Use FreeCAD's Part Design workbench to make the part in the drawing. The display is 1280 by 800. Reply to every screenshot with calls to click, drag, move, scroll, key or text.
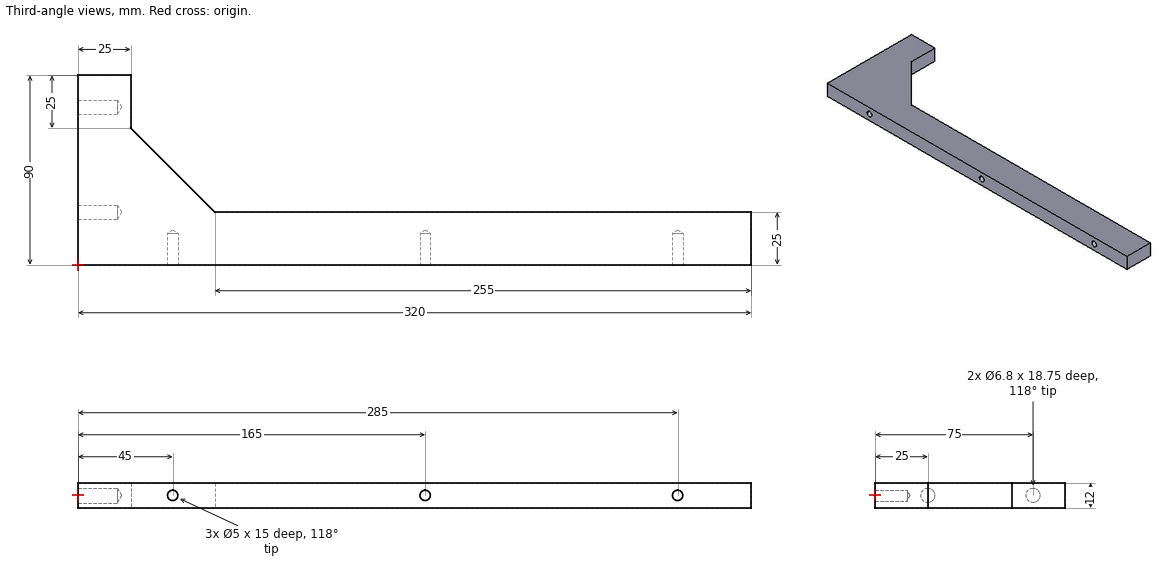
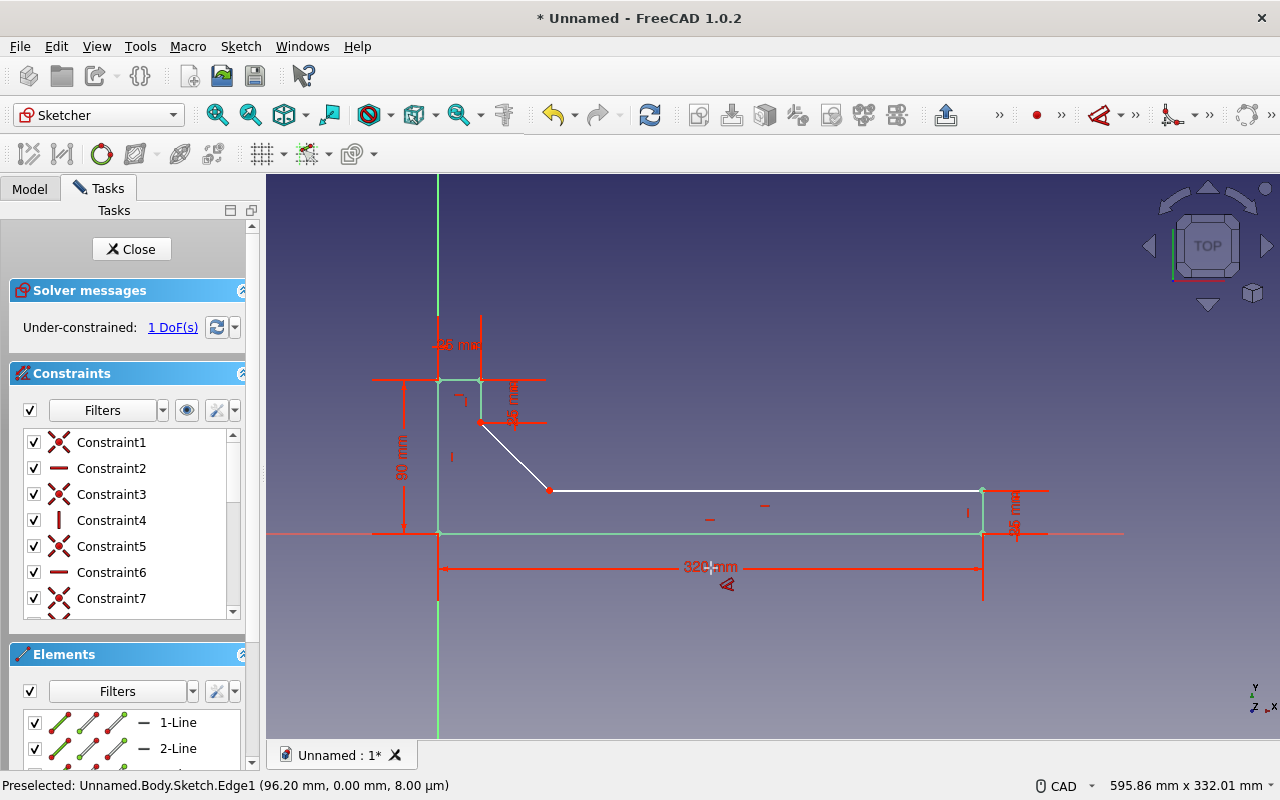
click(853, 491)
click(766, 457)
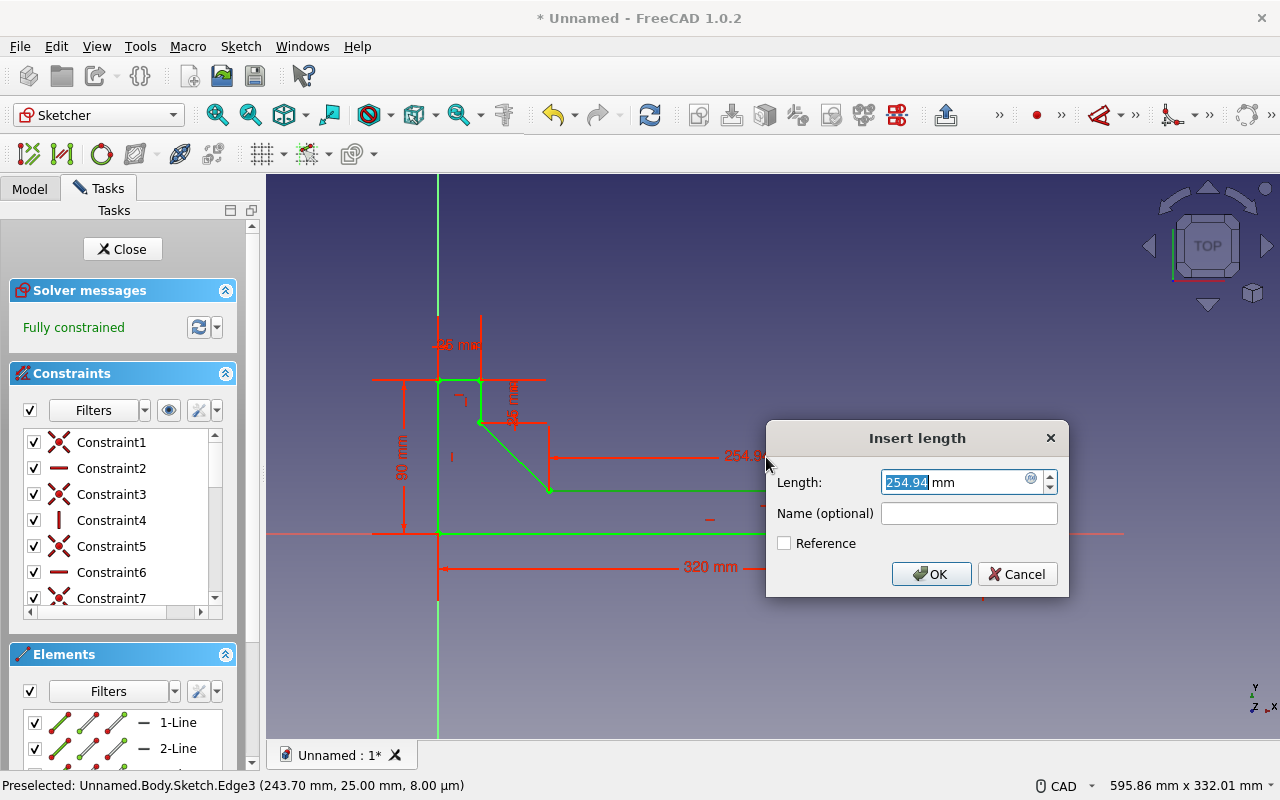
text(255)
key(Return)
key(Escape)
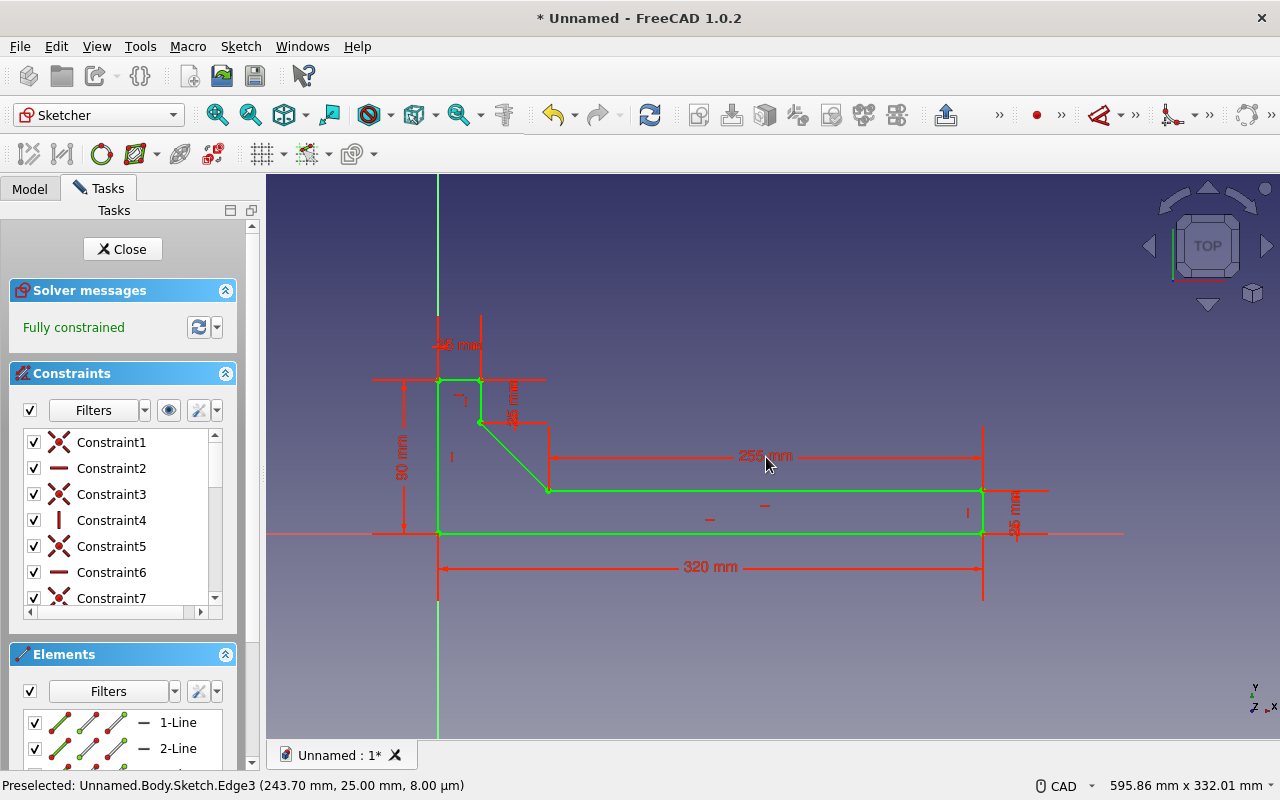
click(123, 249)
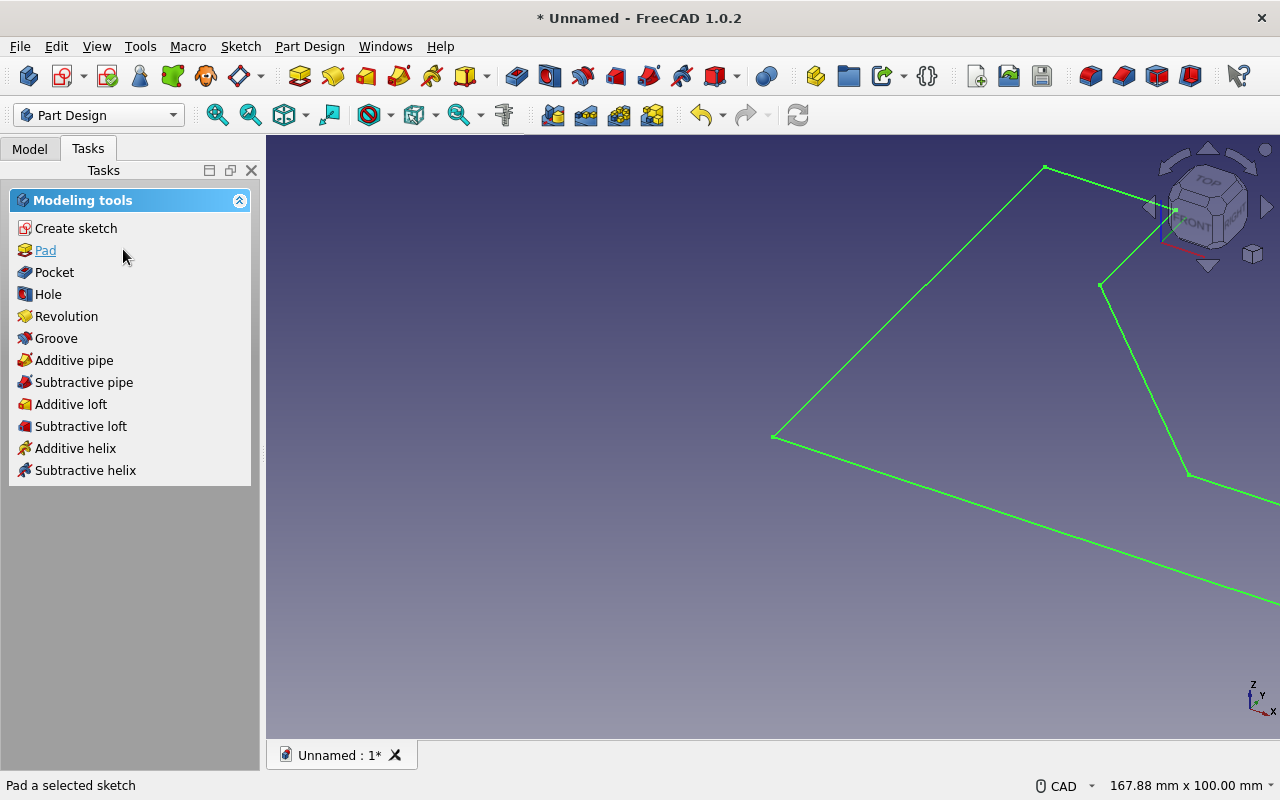
click(300, 76)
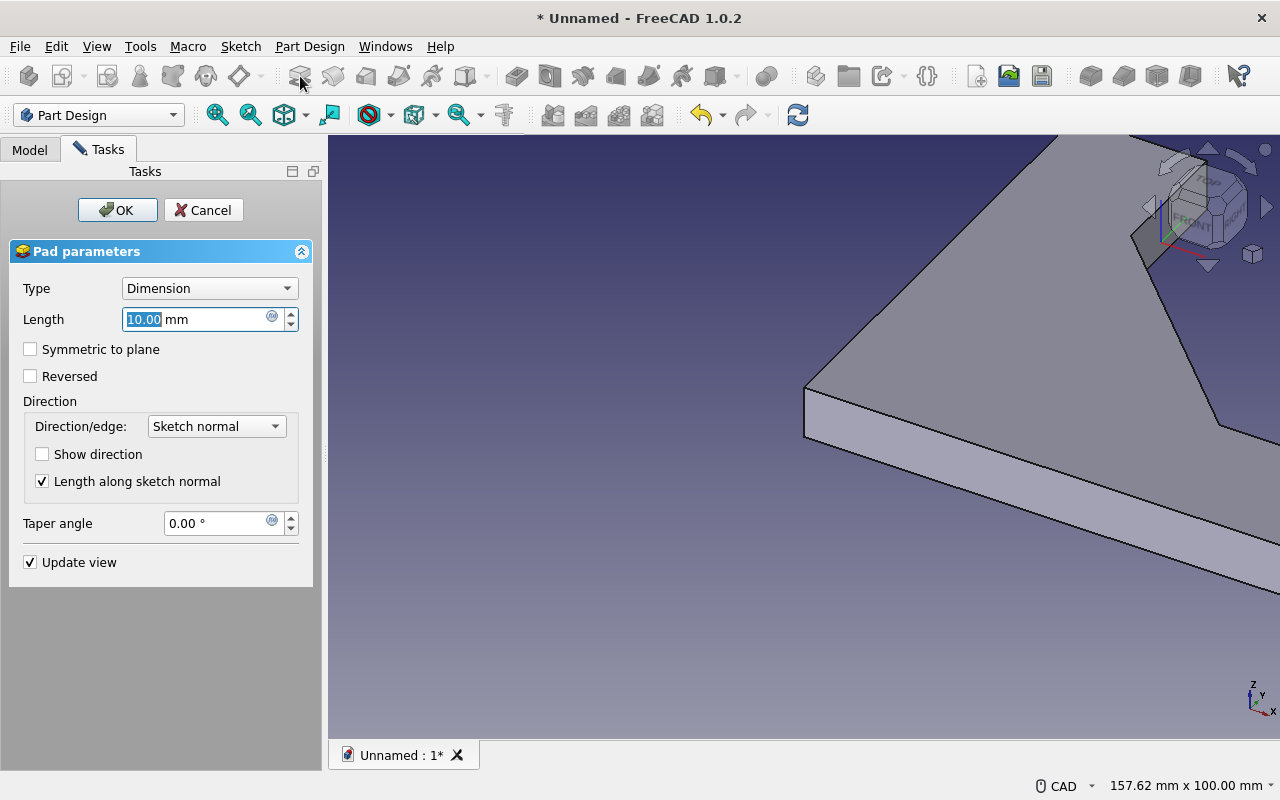
text(12)
key(Tab)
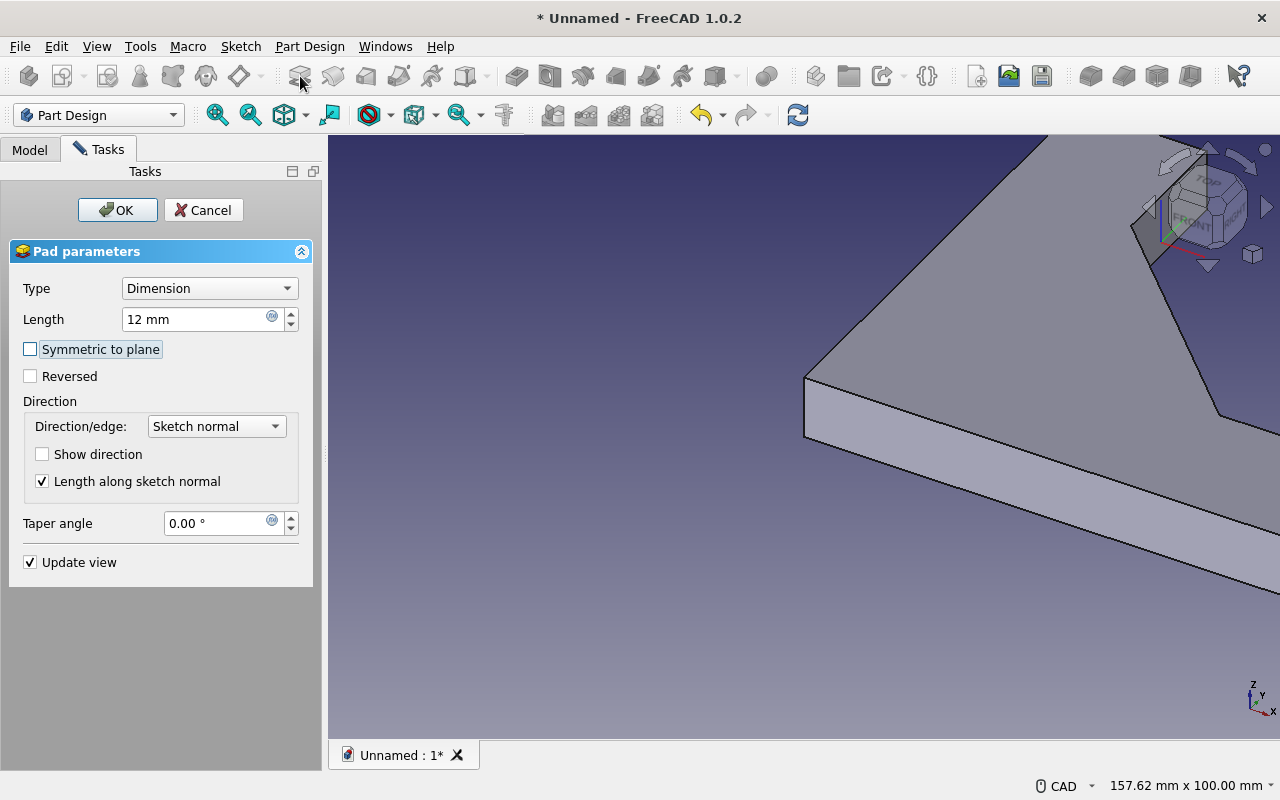
click(31, 349)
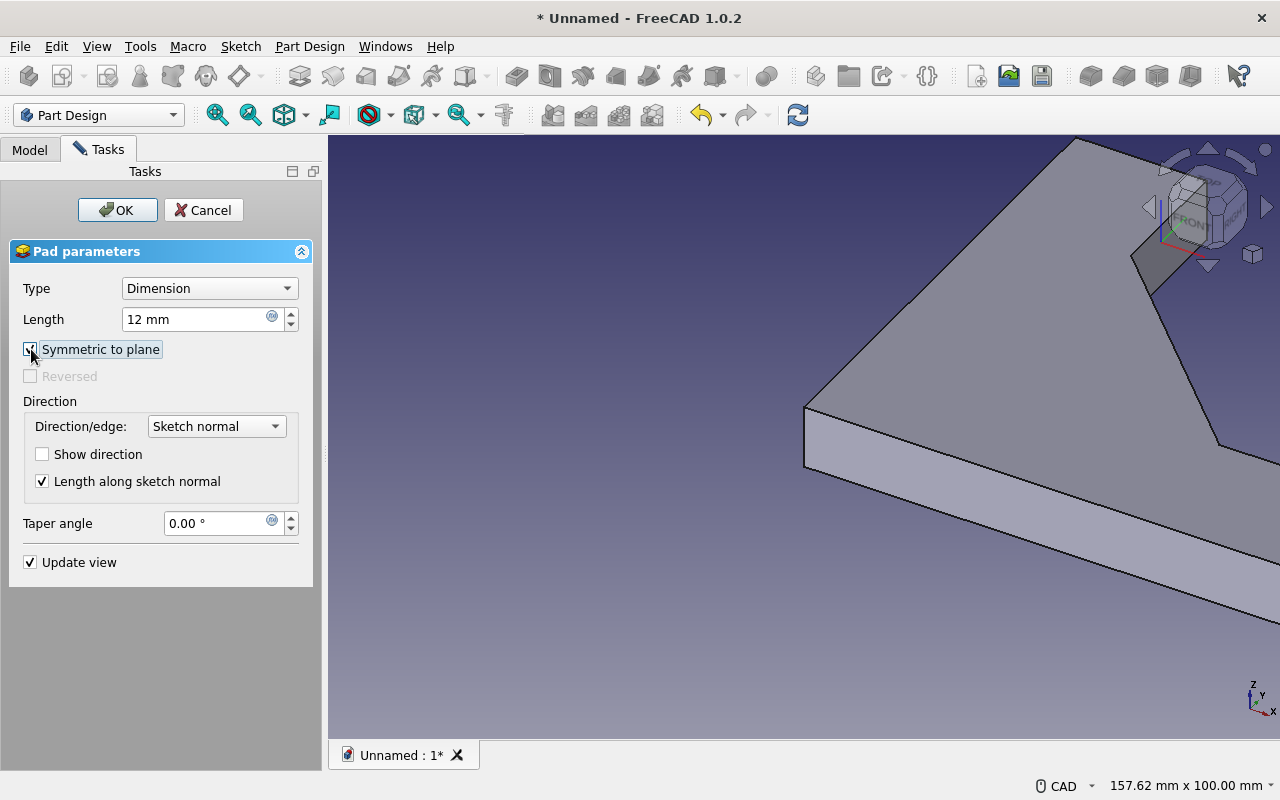
click(118, 210)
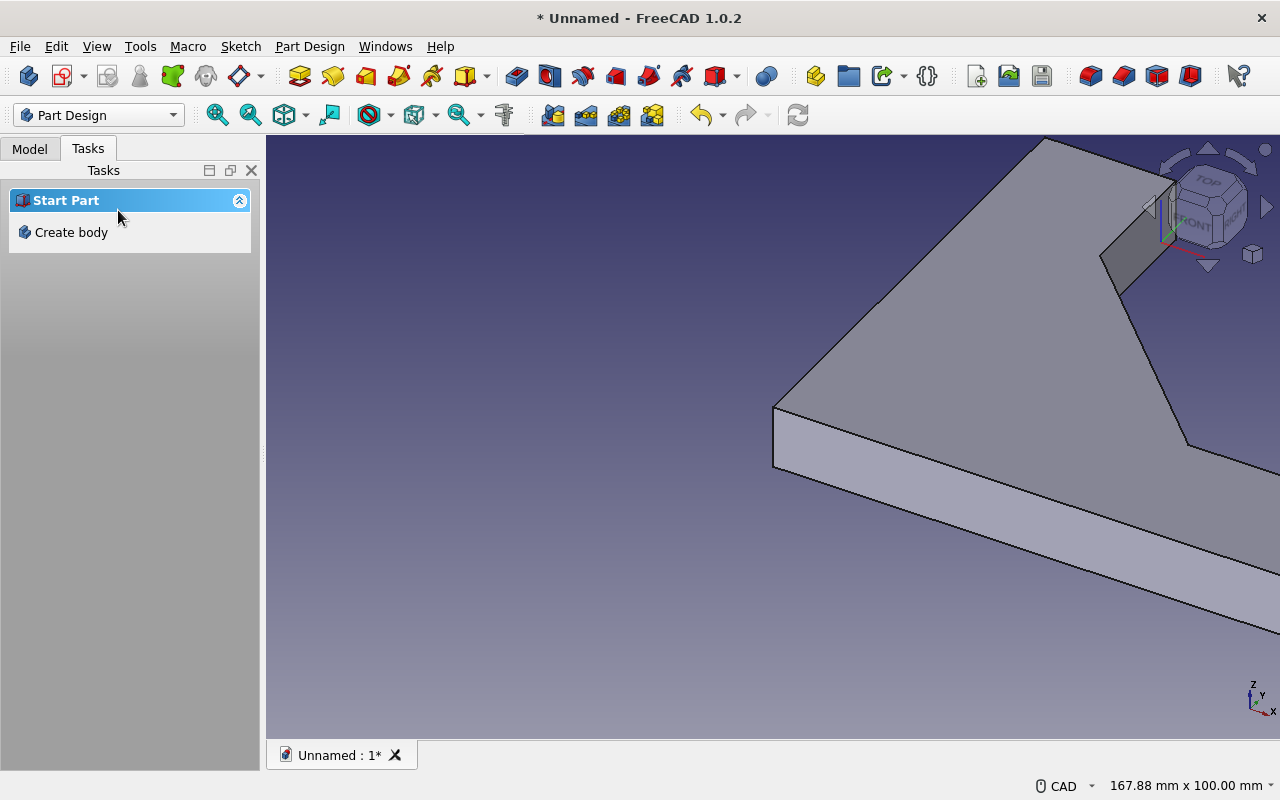
key(v)
key(f)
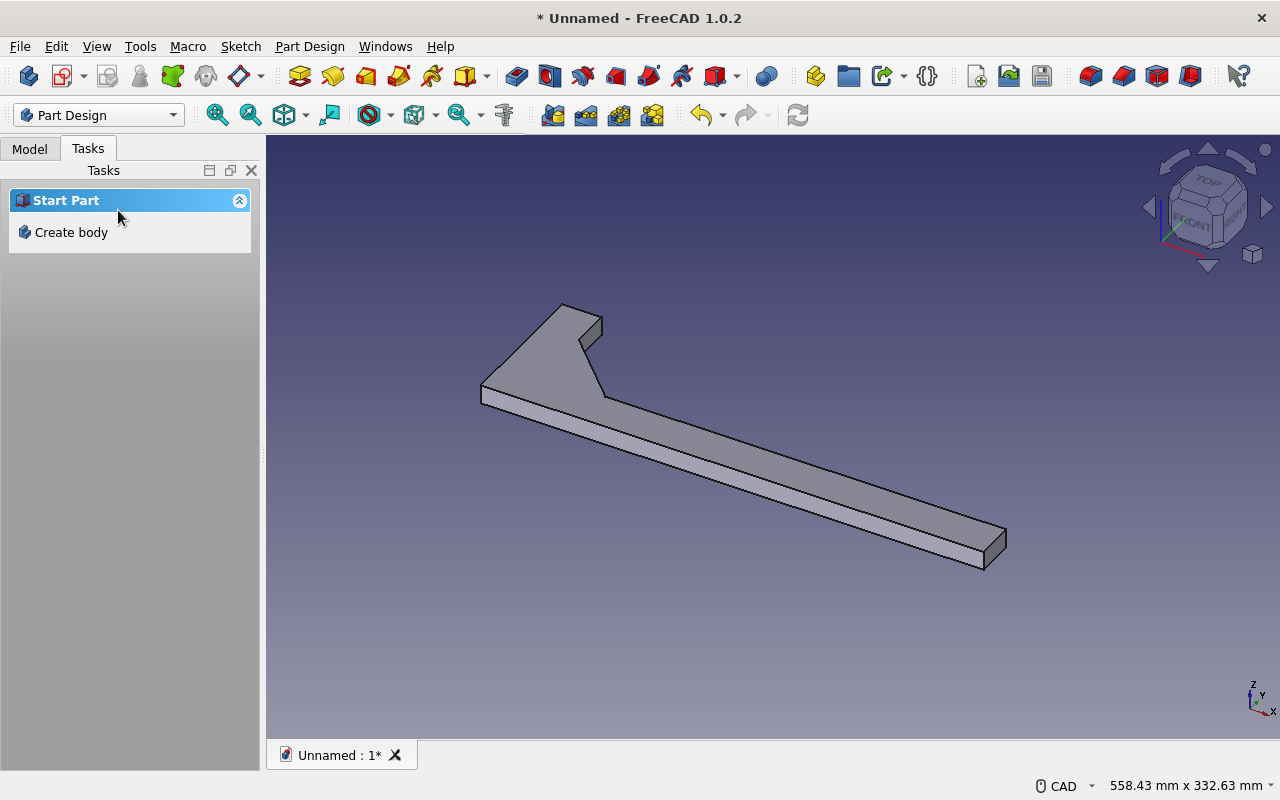
click(62, 76)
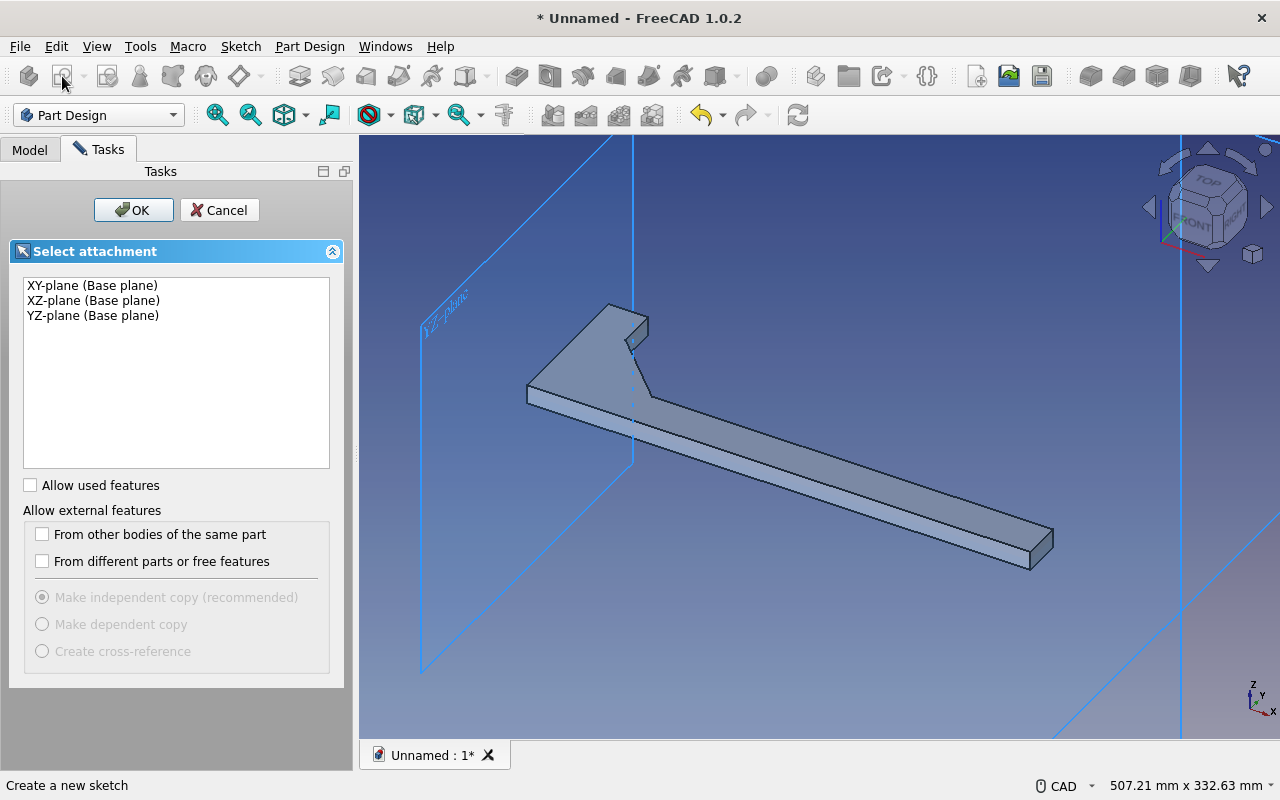
click(84, 316)